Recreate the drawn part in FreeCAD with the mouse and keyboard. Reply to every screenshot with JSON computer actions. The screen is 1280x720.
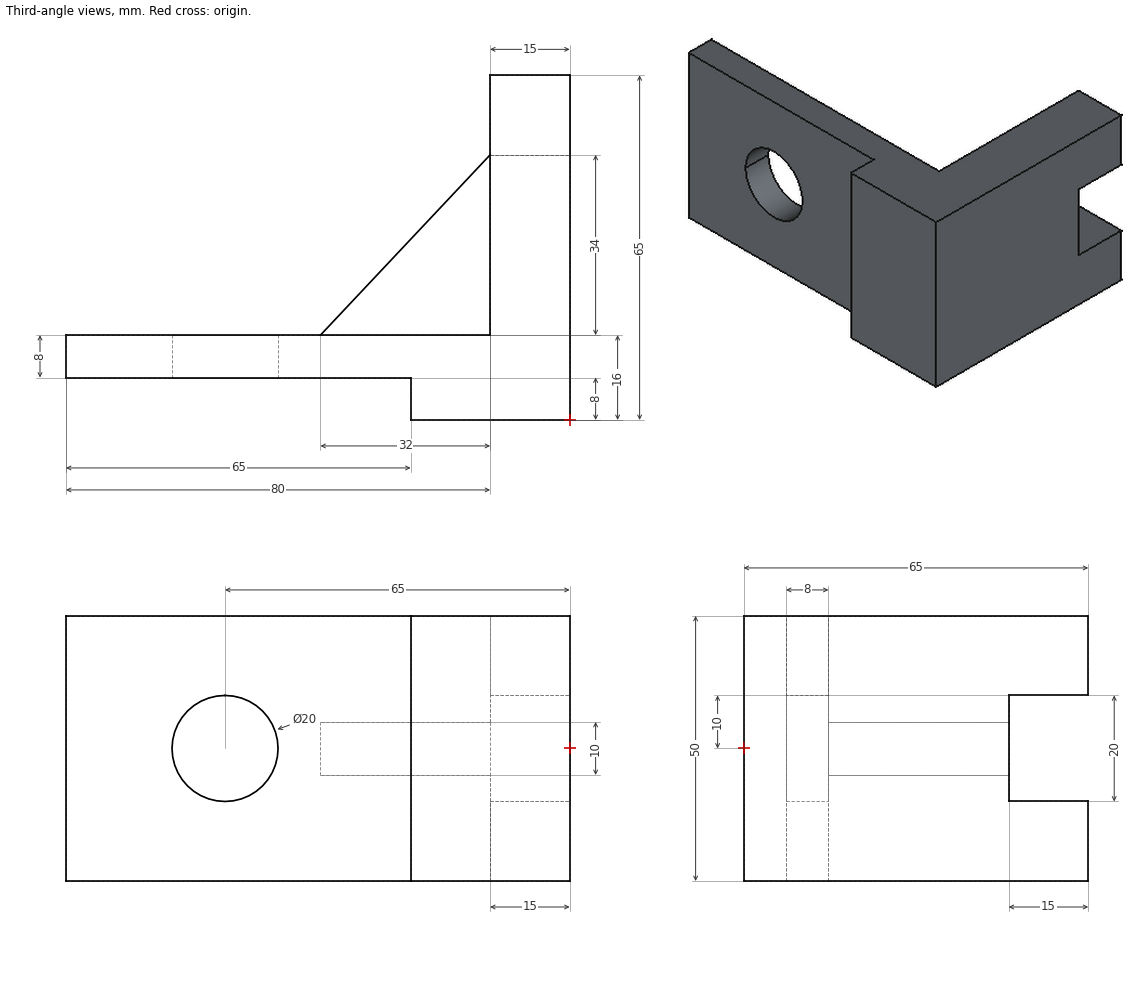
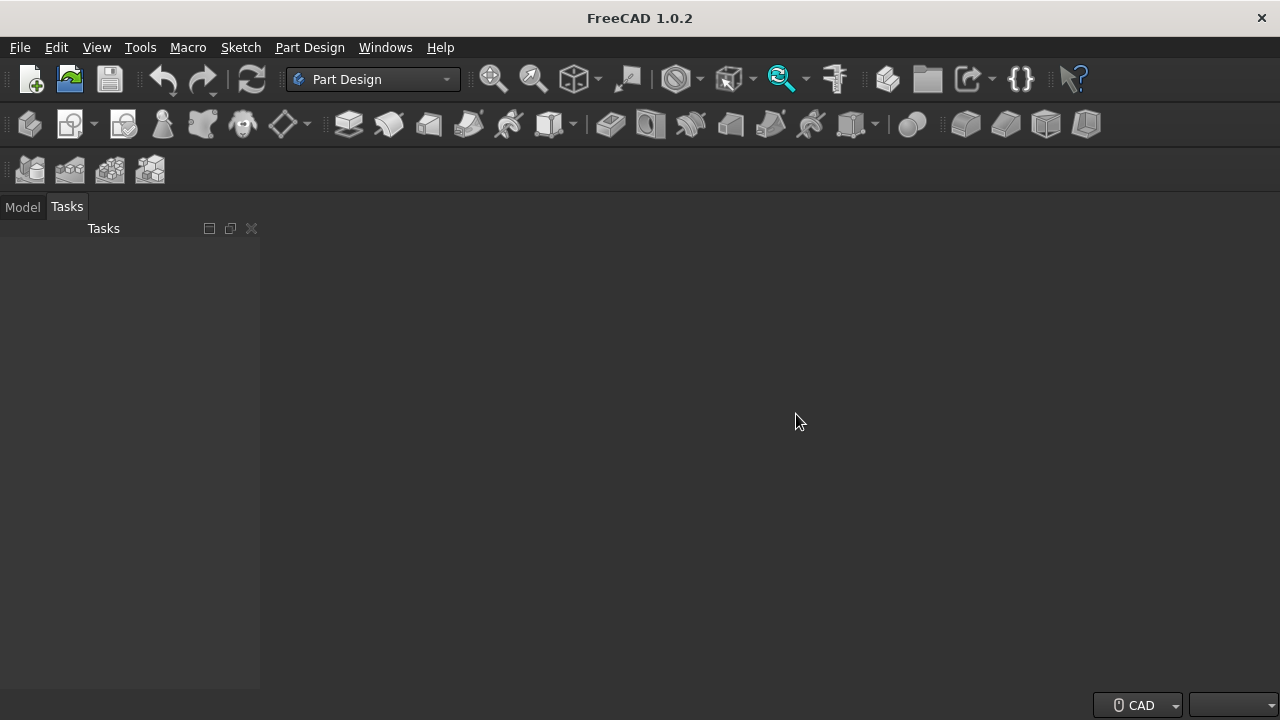
{"action": "left_click", "coordinate": [30, 80]}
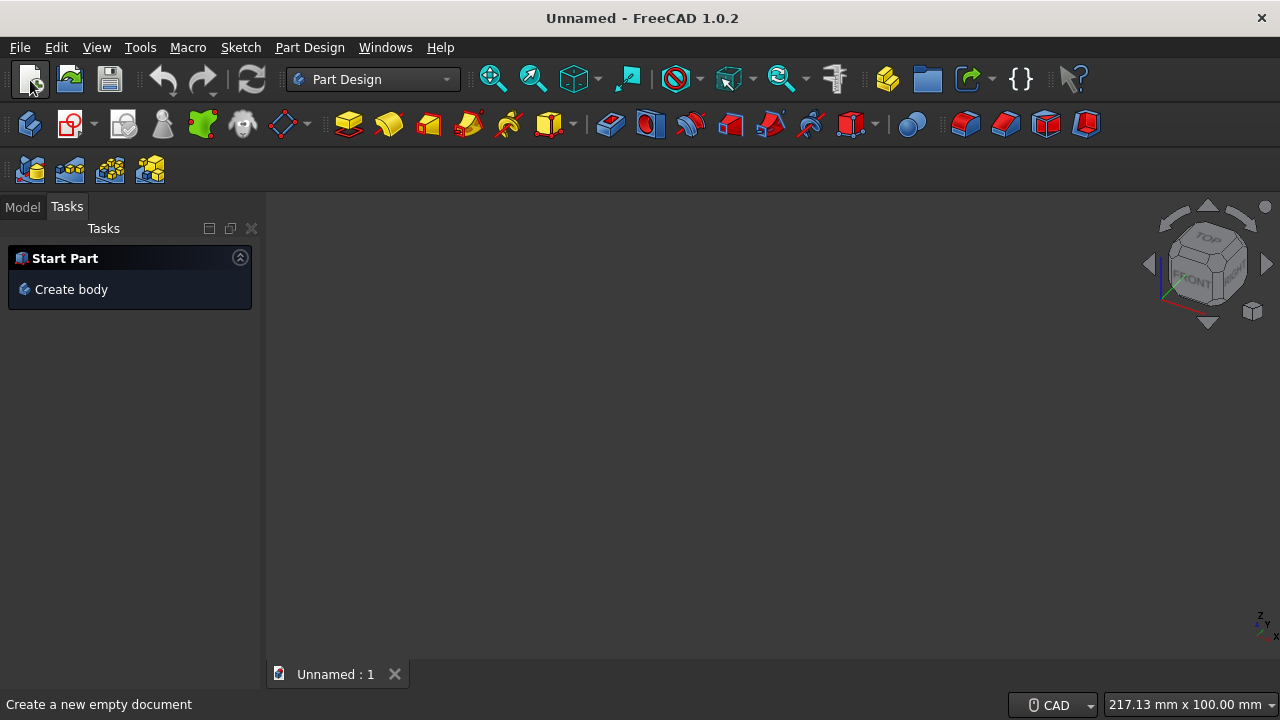
{"action": "left_click", "coordinate": [70, 124]}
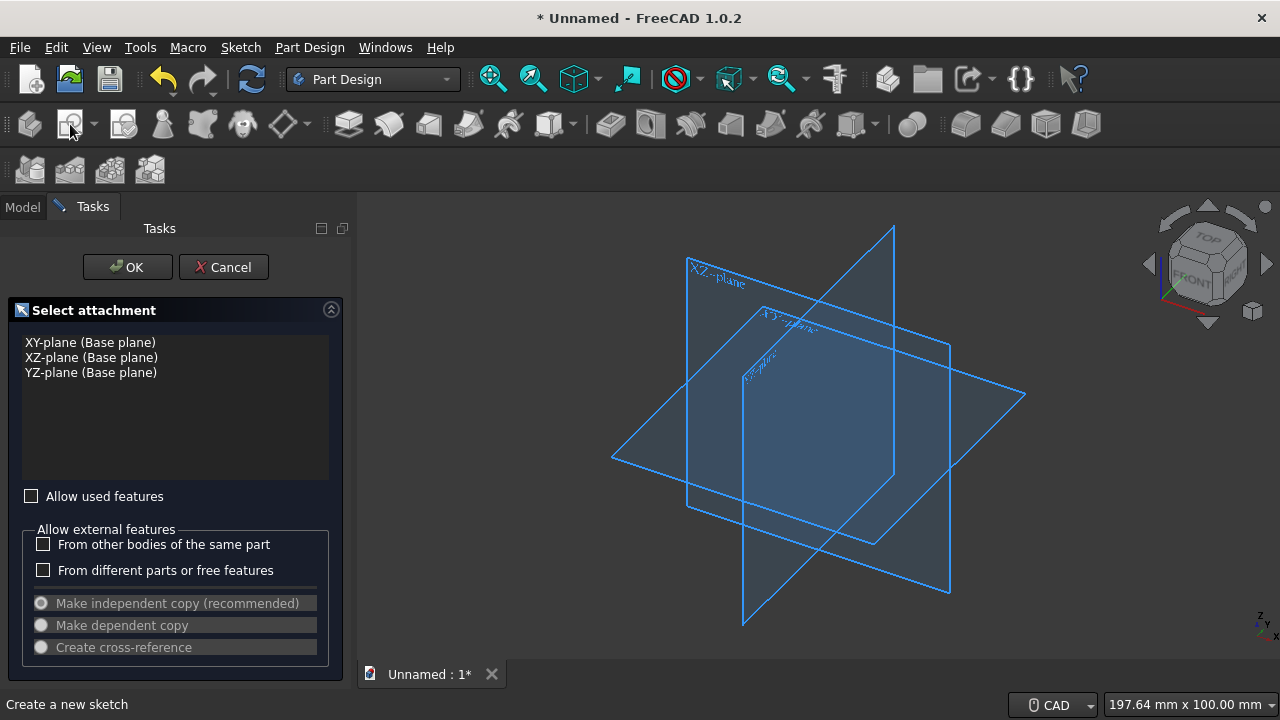
{"action": "left_click", "coordinate": [82, 342]}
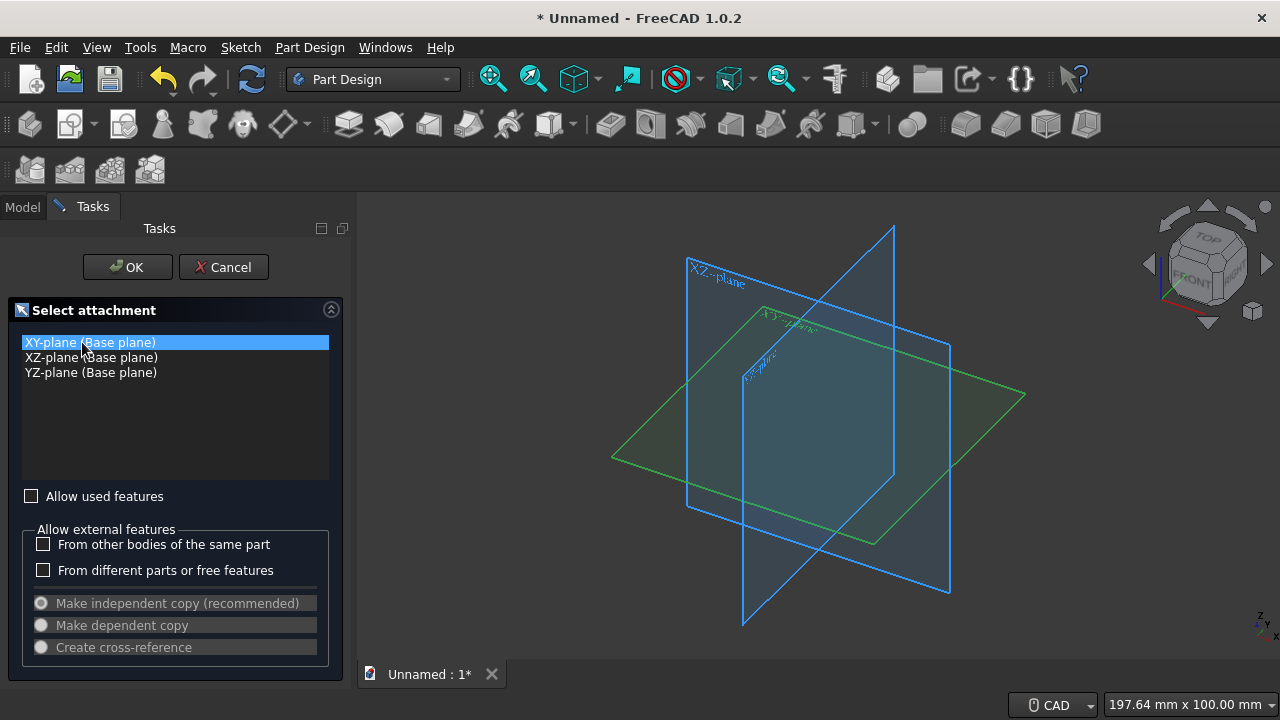
{"action": "left_click", "coordinate": [128, 267]}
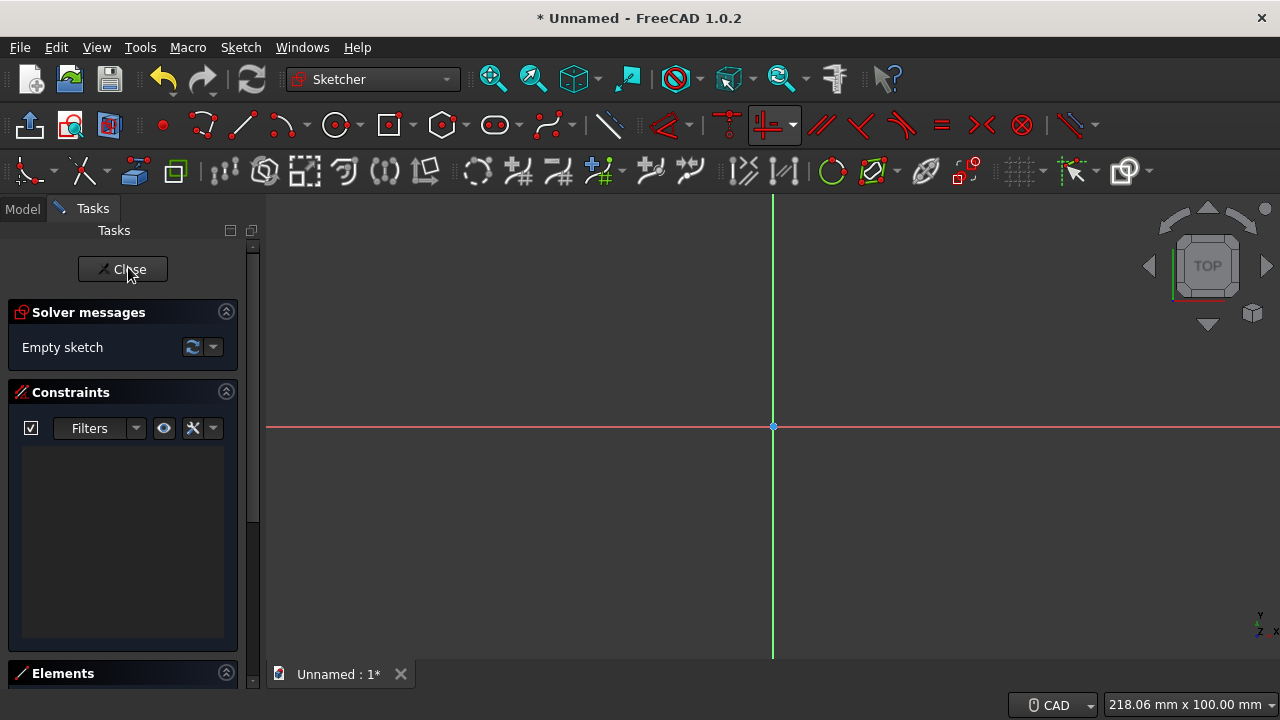
{"action": "scroll", "coordinate": [1014, 631], "scroll_direction": "down", "scroll_amount": 2}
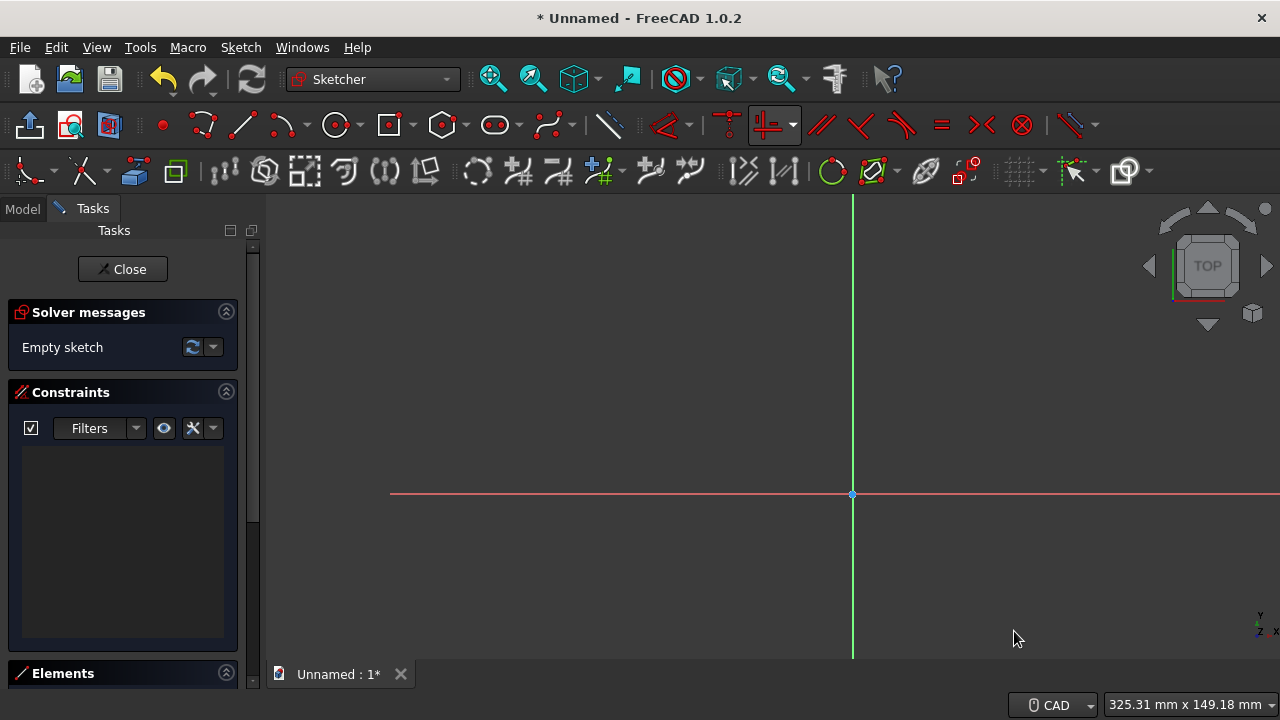
{"action": "scroll", "coordinate": [705, 325], "scroll_direction": "up", "scroll_amount": 2}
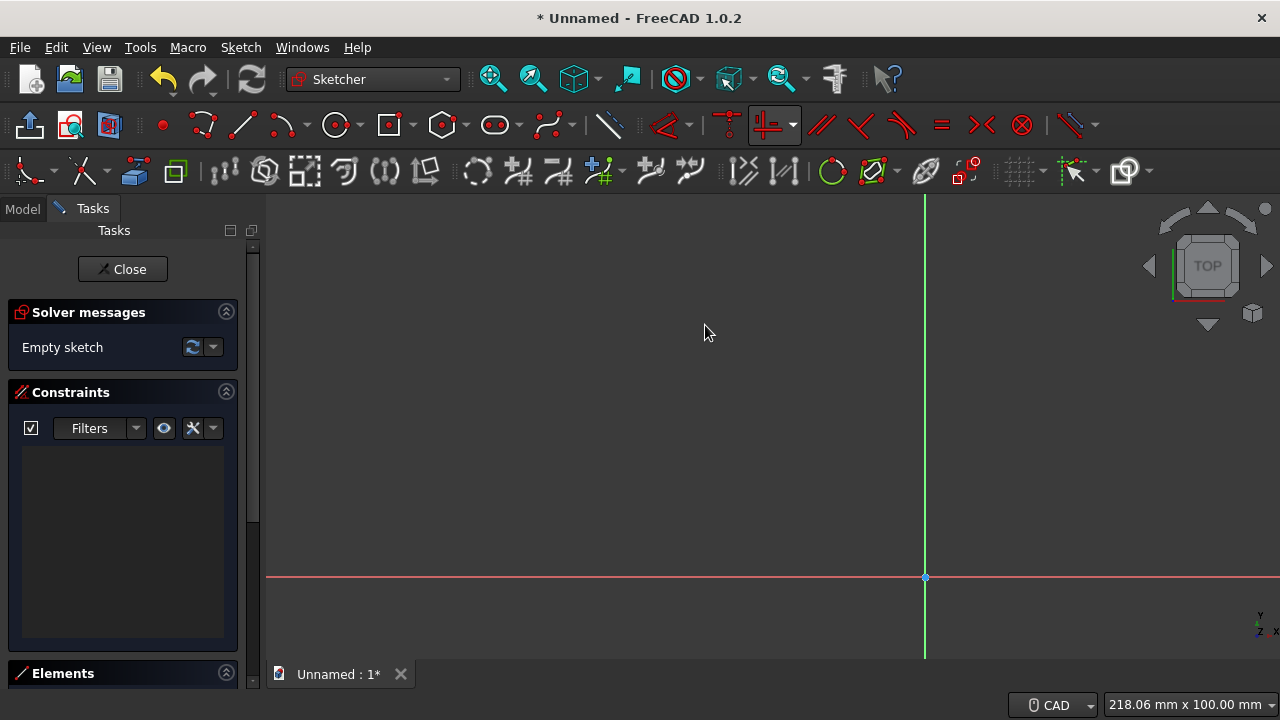
{"action": "left_click", "coordinate": [204, 126]}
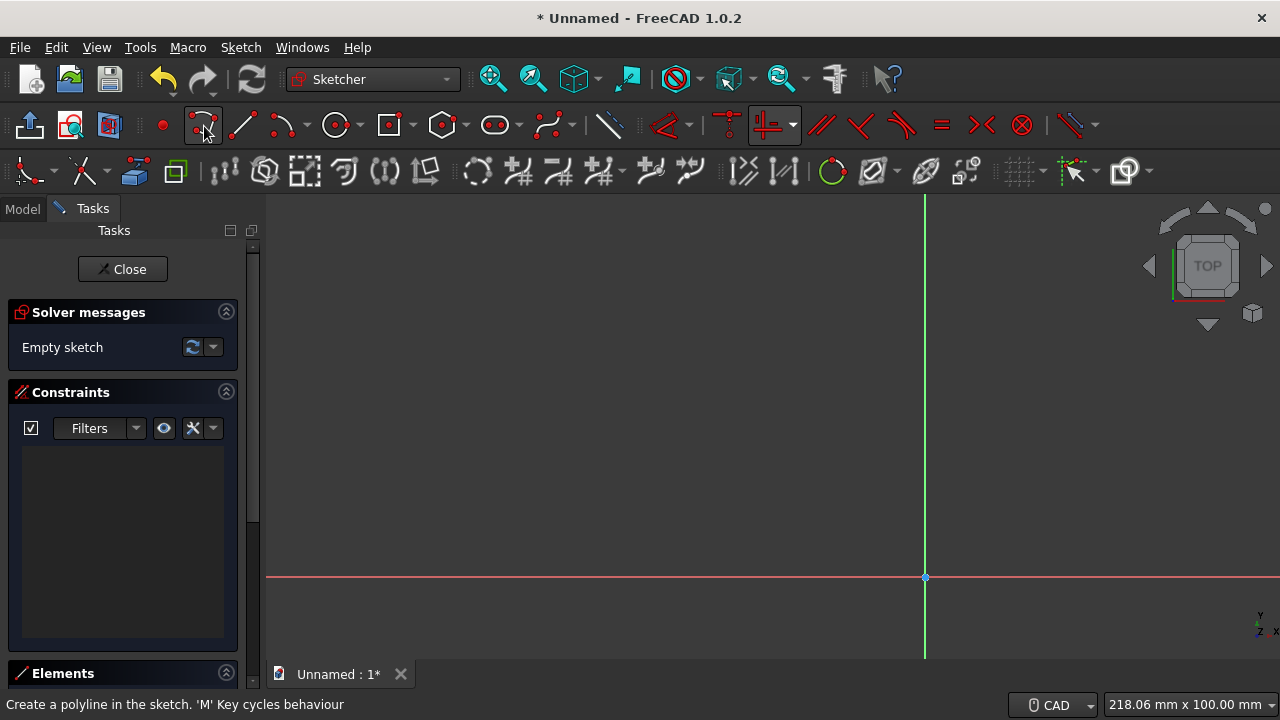
{"action": "left_click", "coordinate": [925, 577]}
{"action": "left_click", "coordinate": [916, 275]}
{"action": "left_click", "coordinate": [855, 275]}
{"action": "left_click", "coordinate": [855, 503]}
{"action": "left_click", "coordinate": [483, 503]}
{"action": "left_click", "coordinate": [483, 540]}
{"action": "left_click", "coordinate": [786, 540]}
{"action": "left_click", "coordinate": [786, 568]}
{"action": "left_click", "coordinate": [925, 577]}
{"action": "key", "text": "Escape"}
{"action": "key", "text": "Escape"}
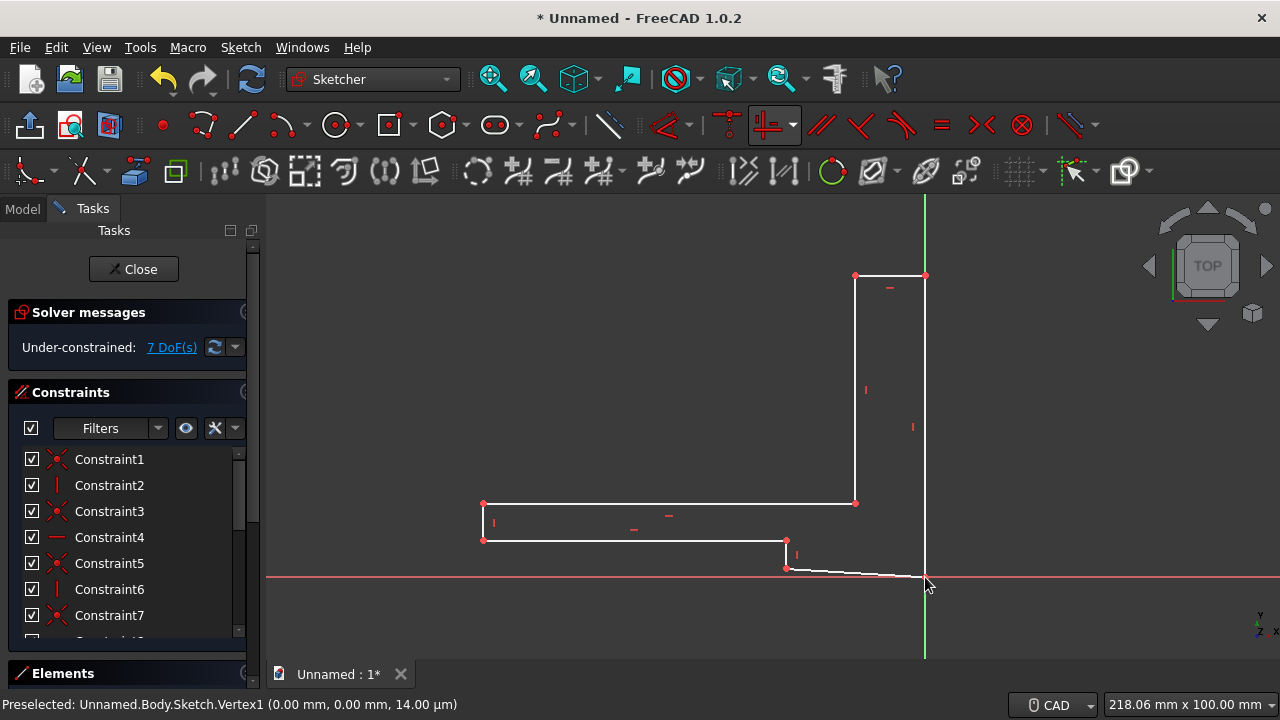
{"action": "left_click", "coordinate": [883, 575]}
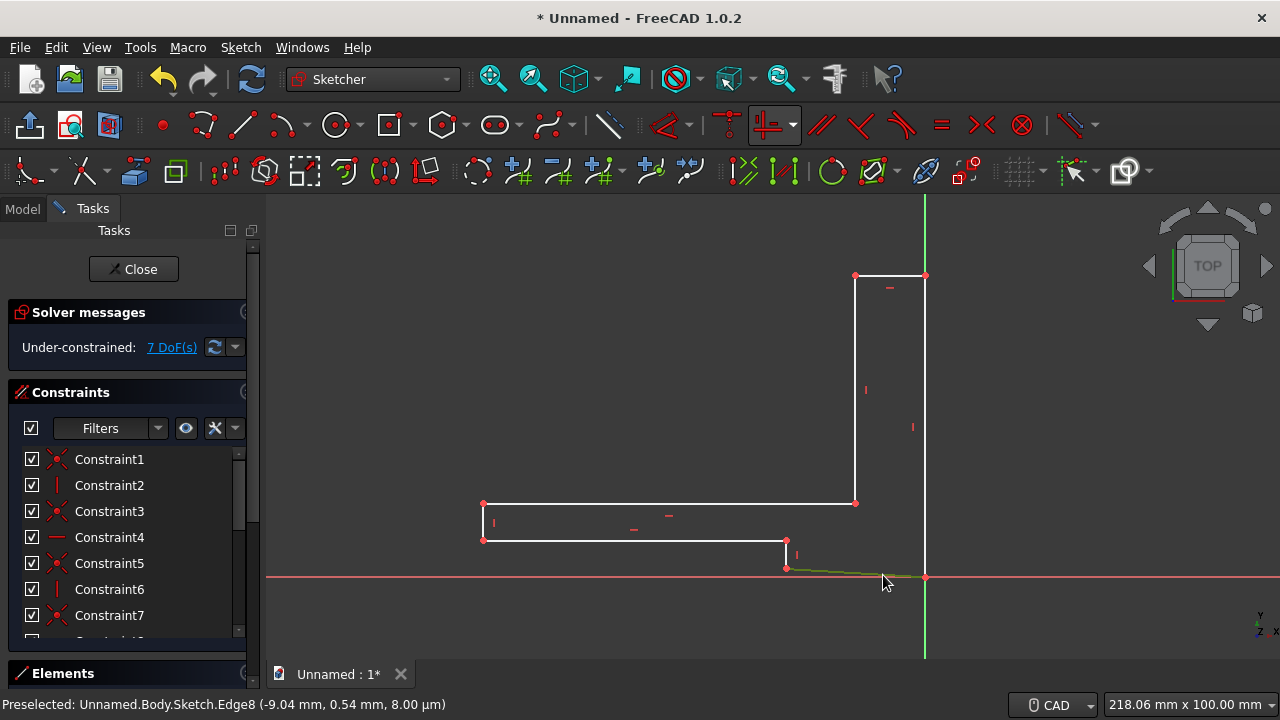
{"action": "key", "text": "h"}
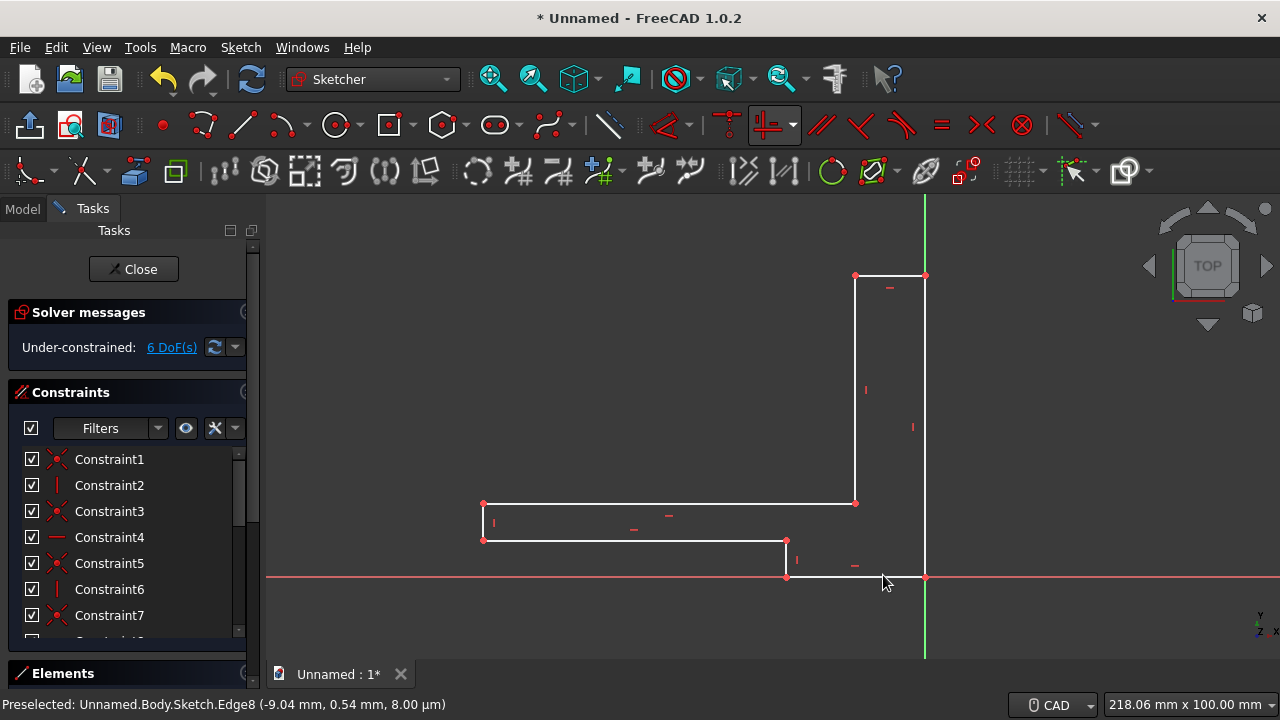
{"action": "key", "text": "d"}